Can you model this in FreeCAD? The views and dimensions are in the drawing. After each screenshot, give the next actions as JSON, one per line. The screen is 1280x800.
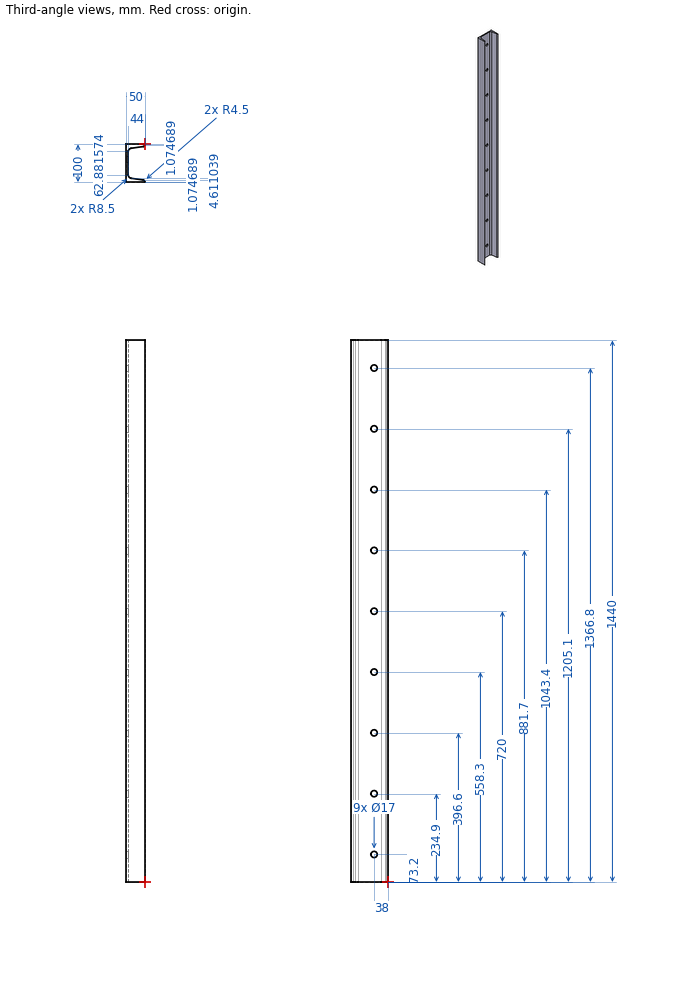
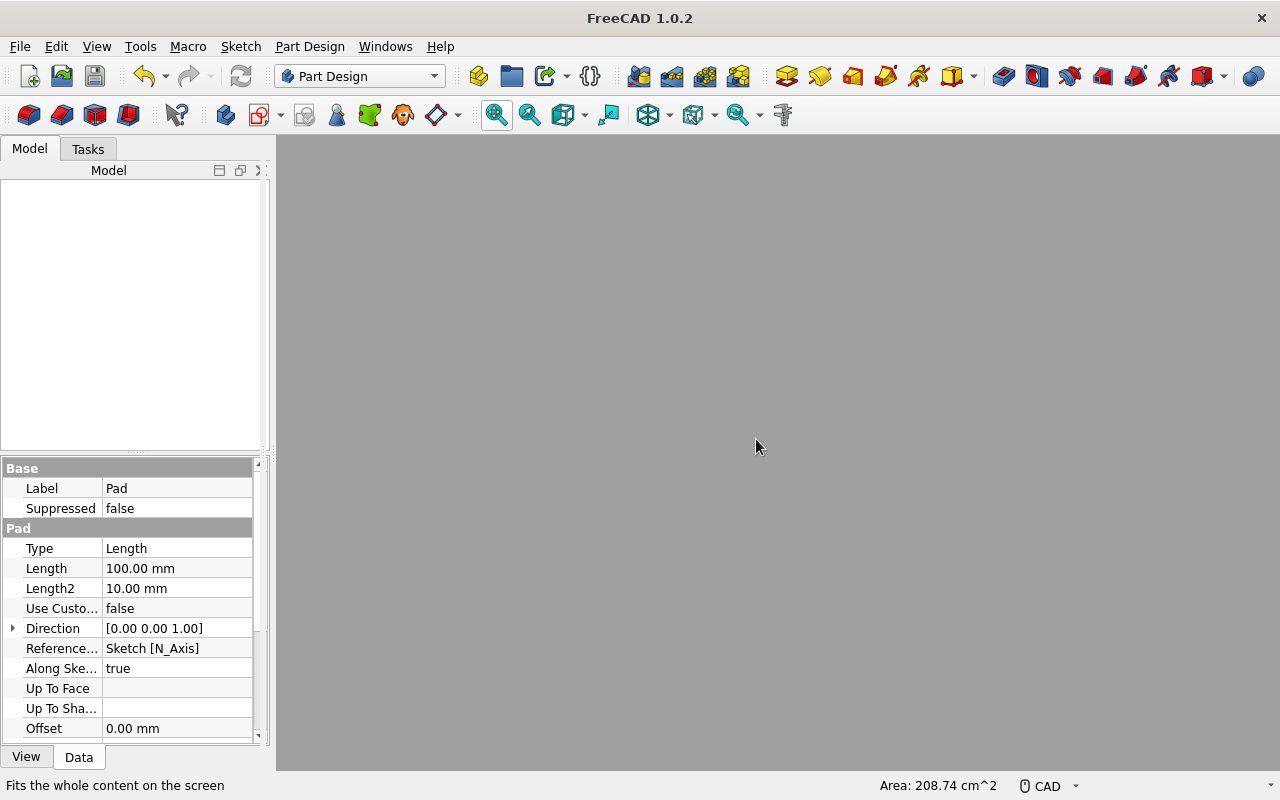
{"action": "left_click", "coordinate": [29, 76]}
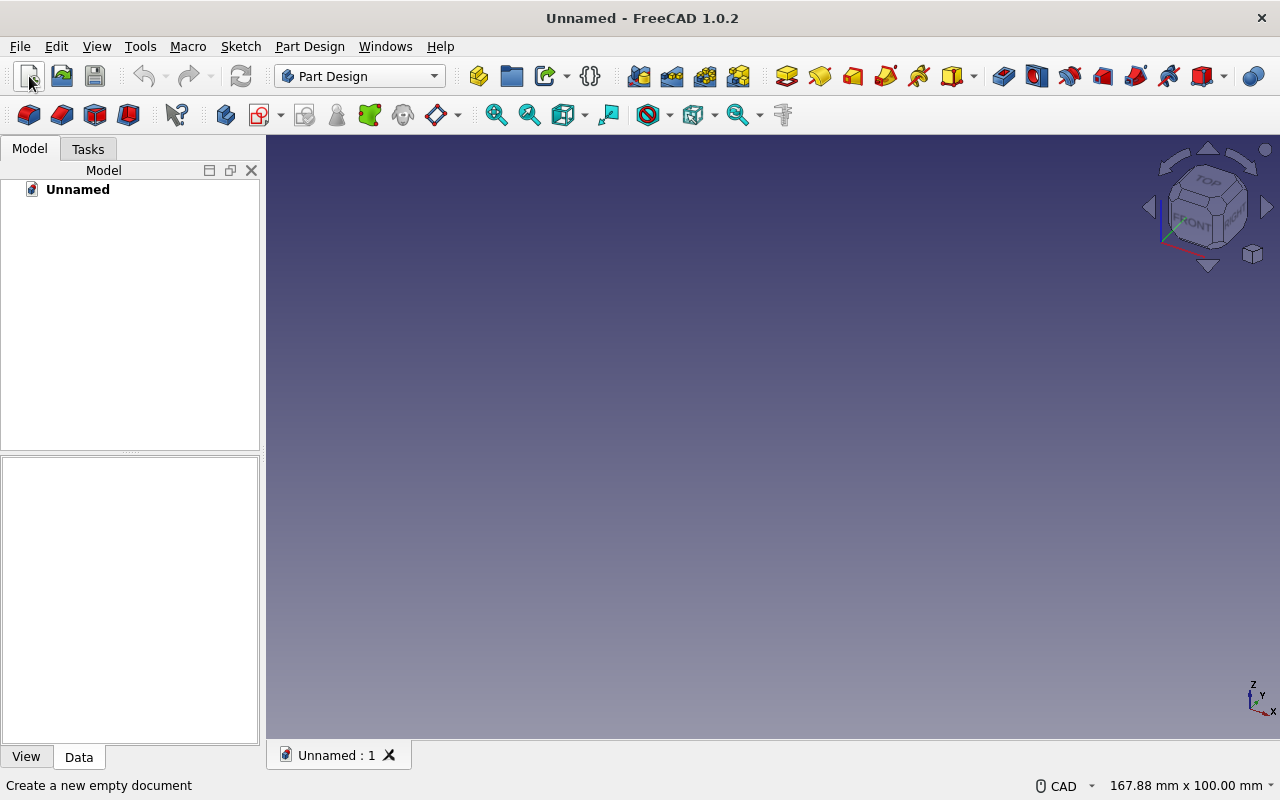
{"action": "left_click", "coordinate": [258, 116]}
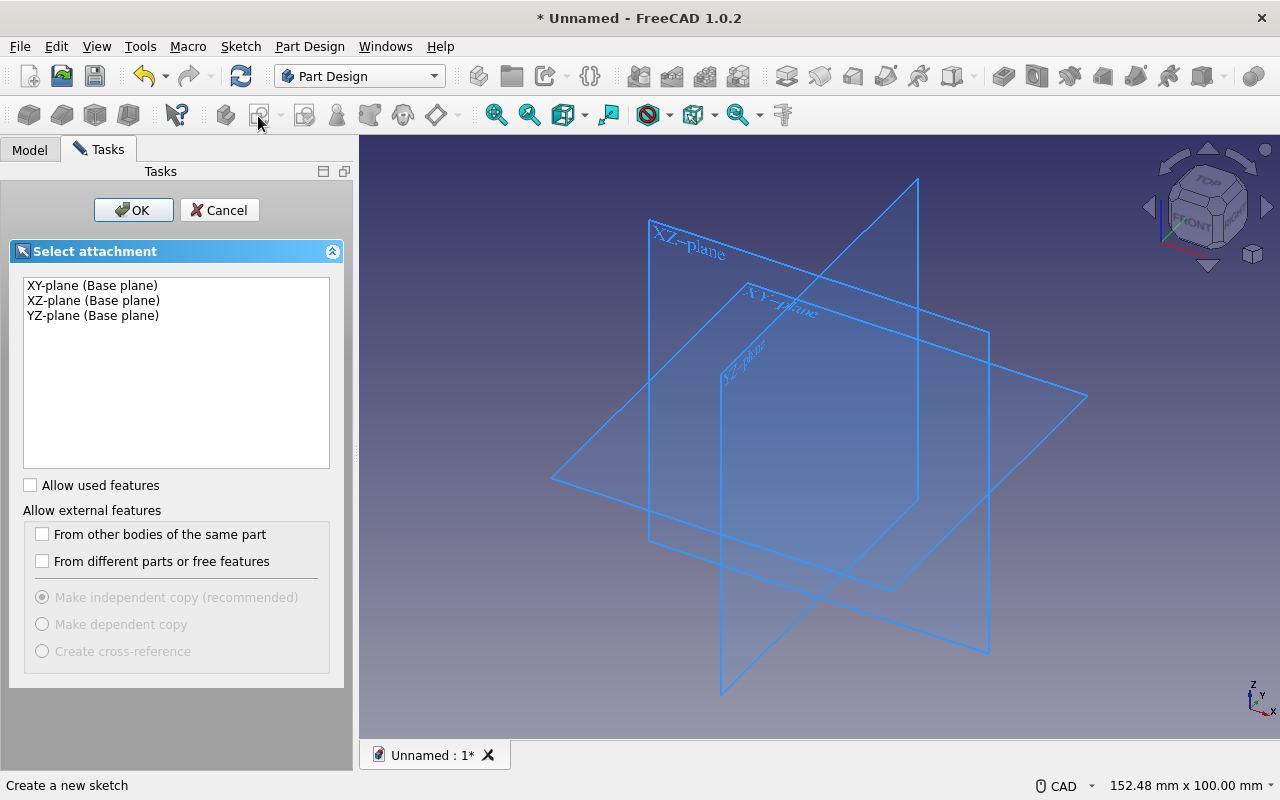
{"action": "left_click", "coordinate": [84, 286]}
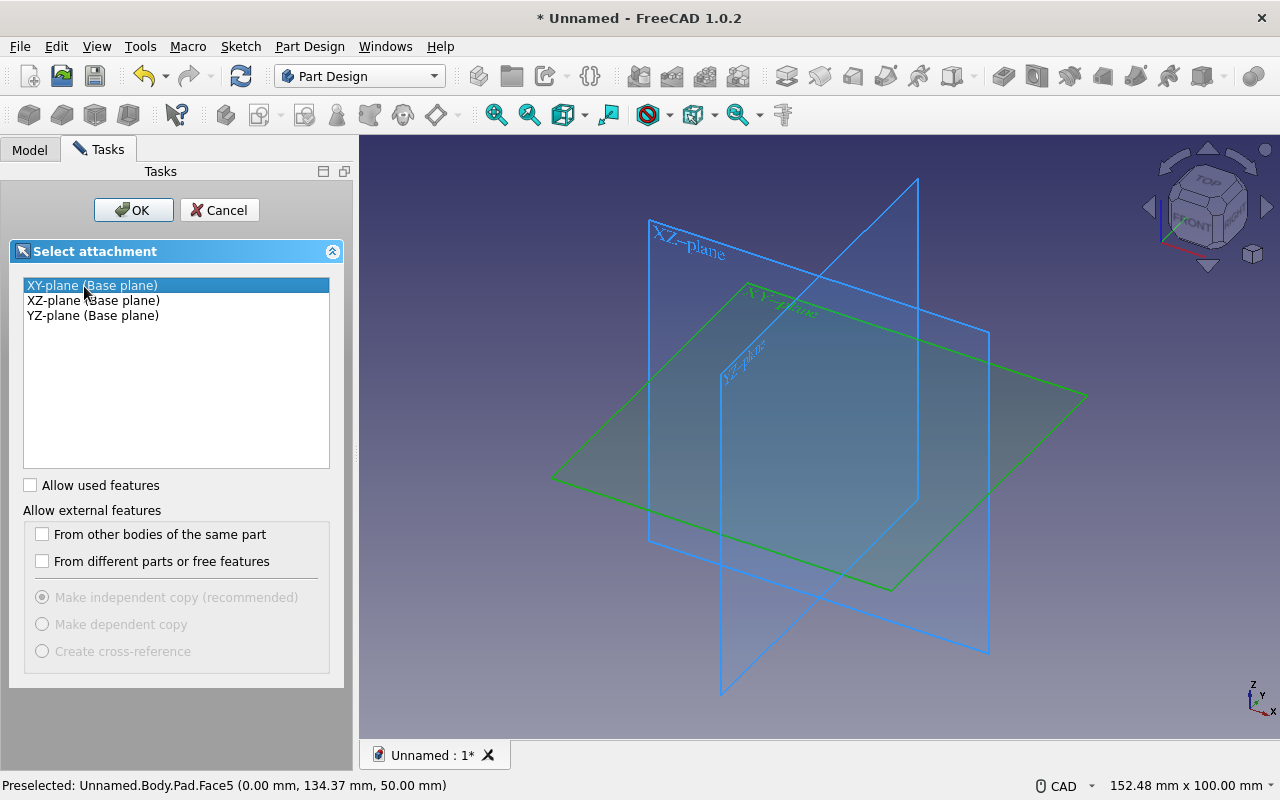
{"action": "left_click", "coordinate": [134, 210]}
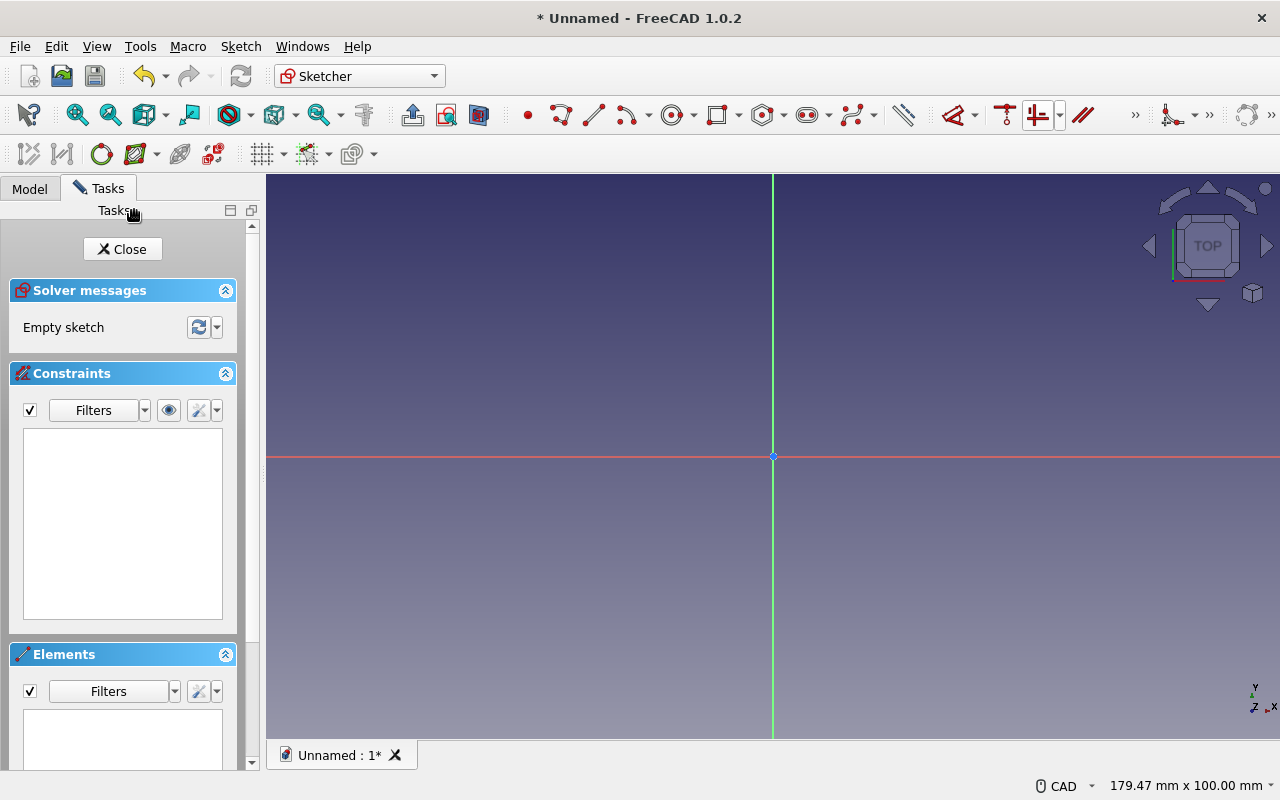
{"action": "scroll", "coordinate": [793, 202], "scroll_direction": "down", "scroll_amount": 3}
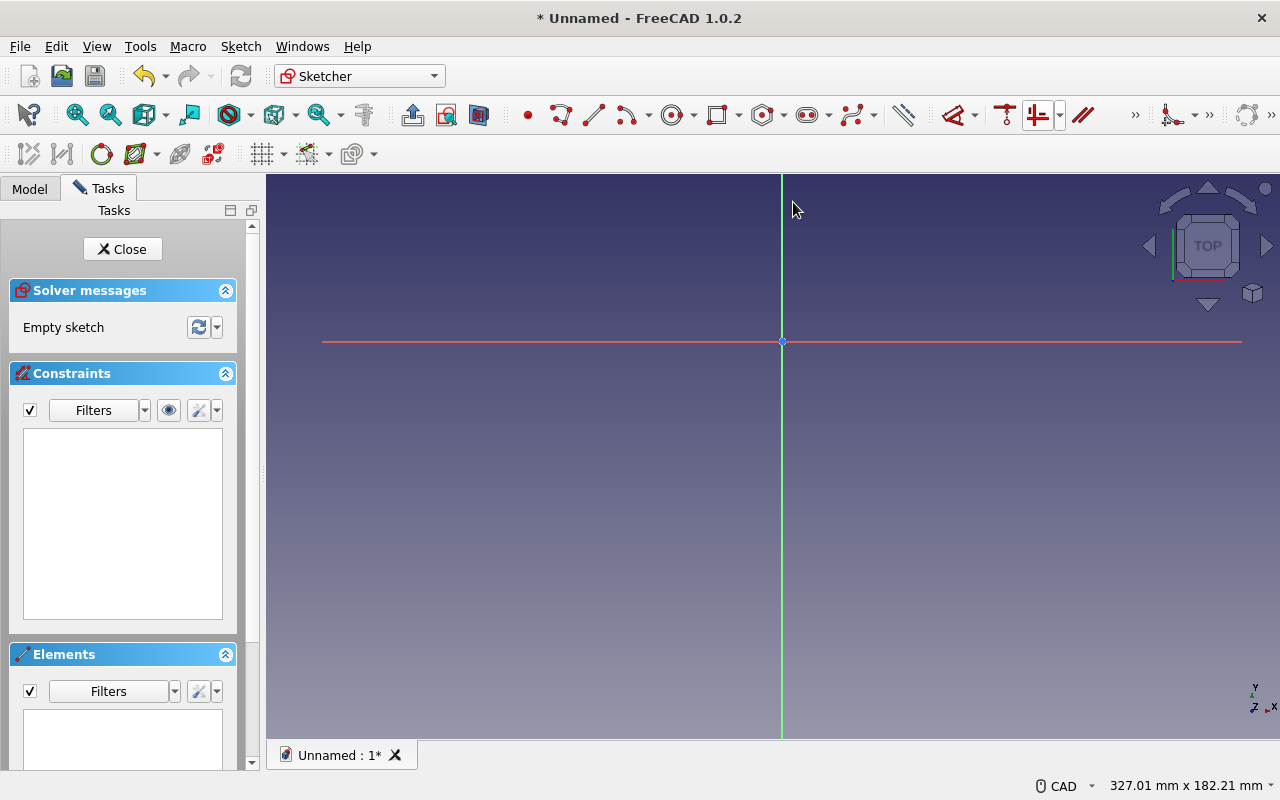
{"action": "left_click", "coordinate": [594, 116]}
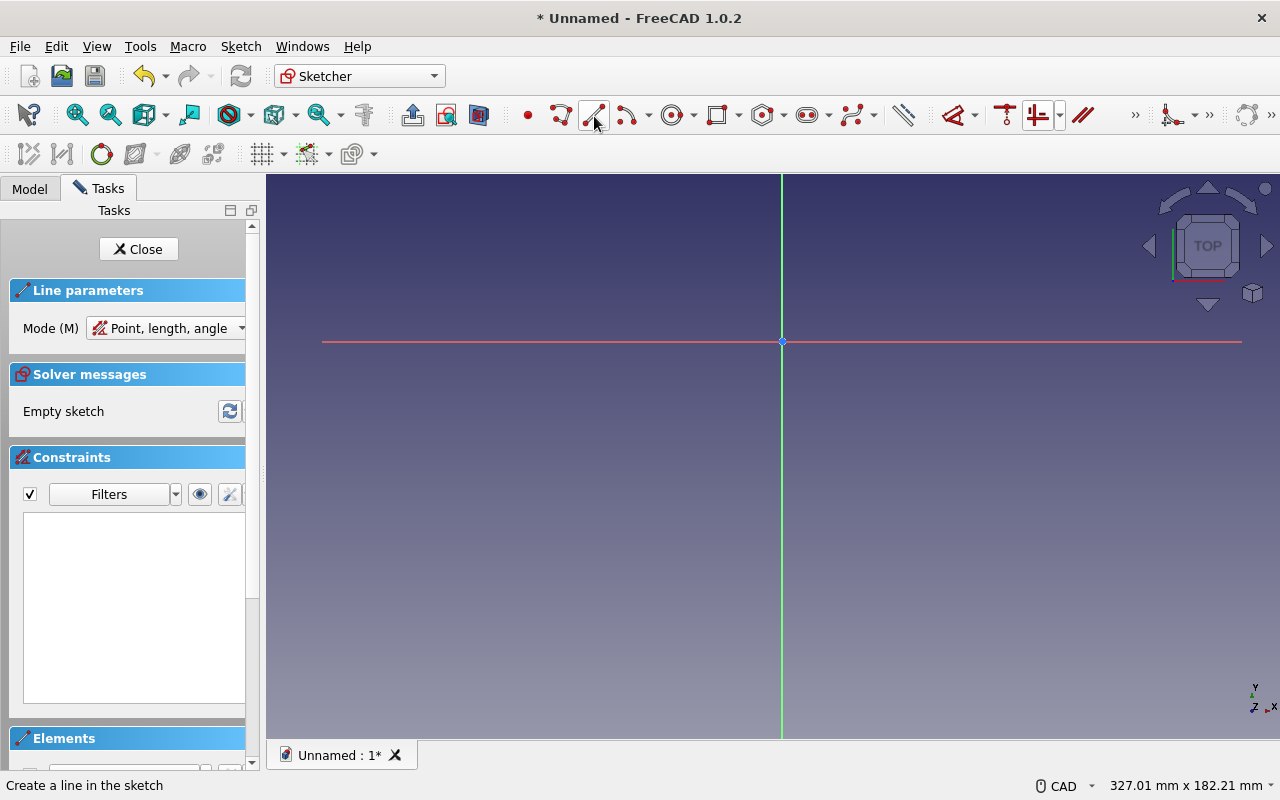
{"action": "scroll", "coordinate": [770, 635], "scroll_direction": "up", "scroll_amount": 2}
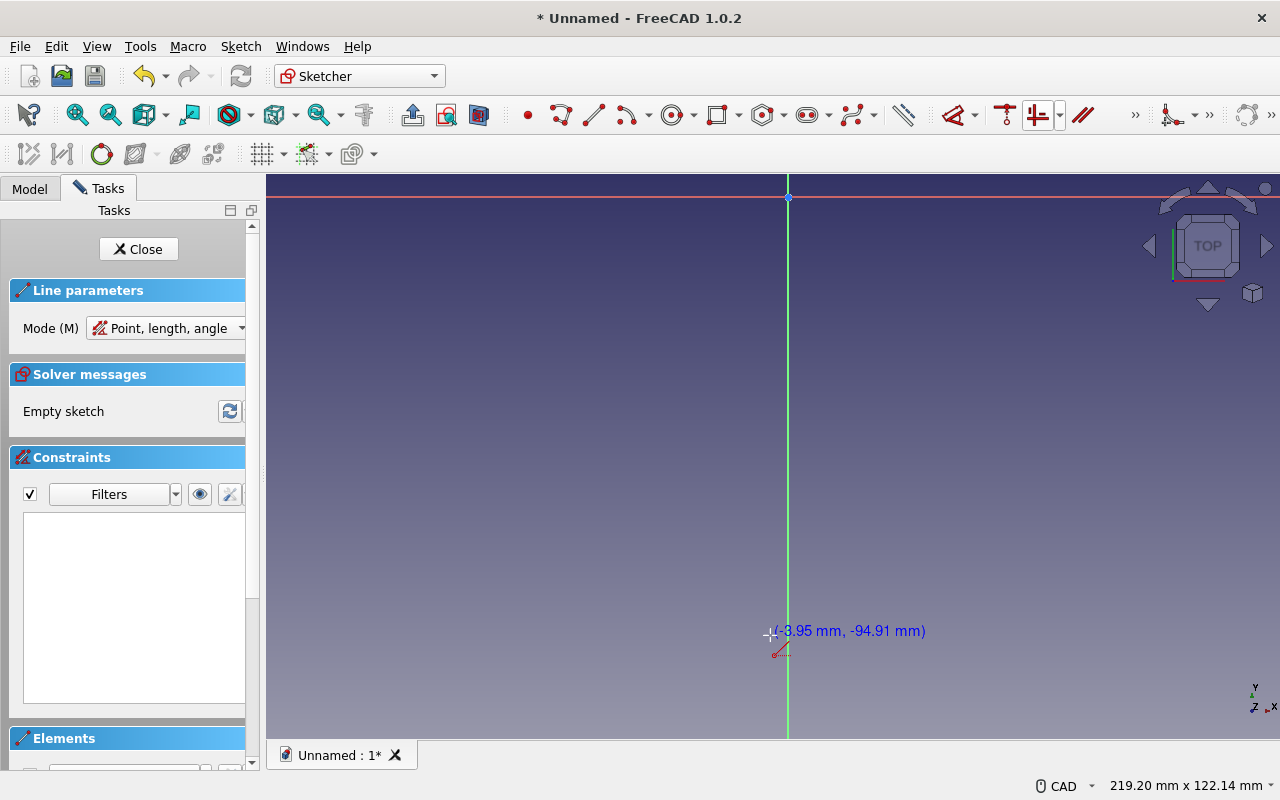
{"action": "left_click", "coordinate": [770, 634]}
{"action": "left_click", "coordinate": [618, 613]}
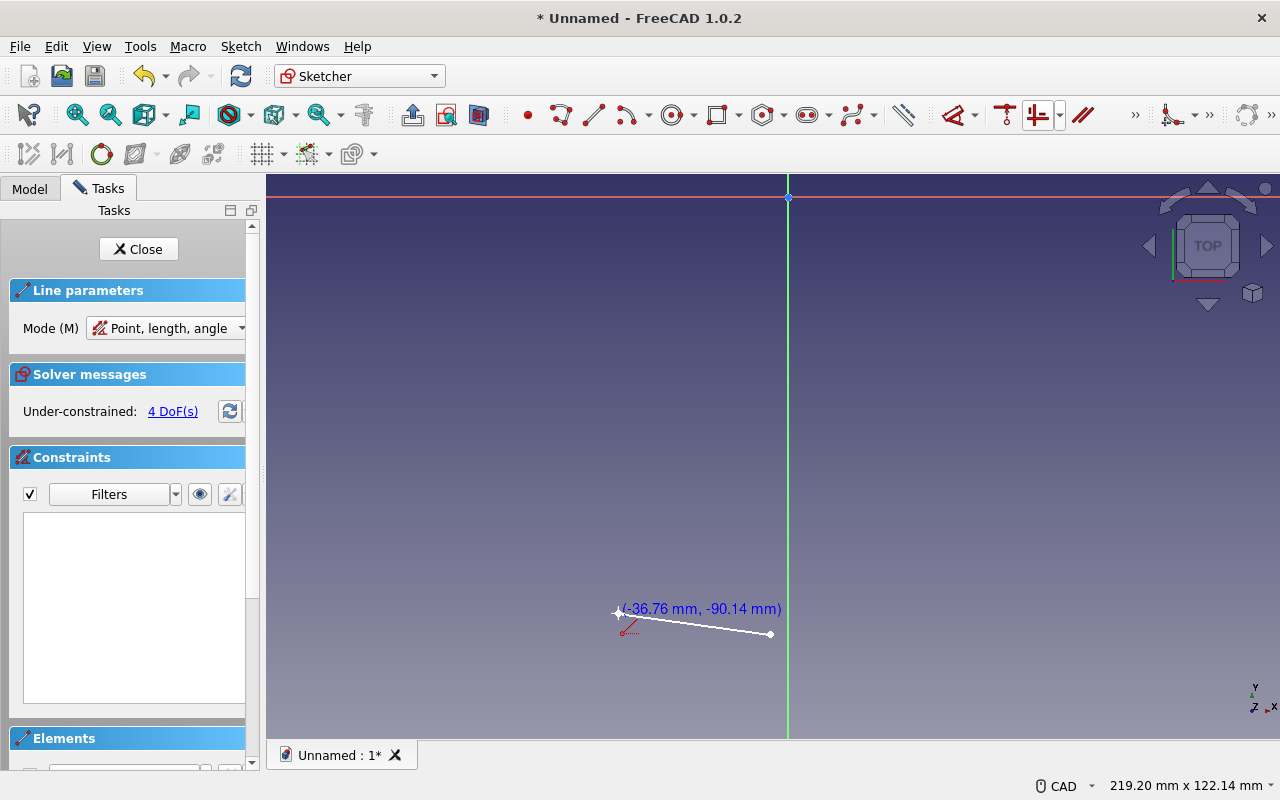
{"action": "left_click", "coordinate": [585, 574]}
{"action": "left_click", "coordinate": [585, 283]}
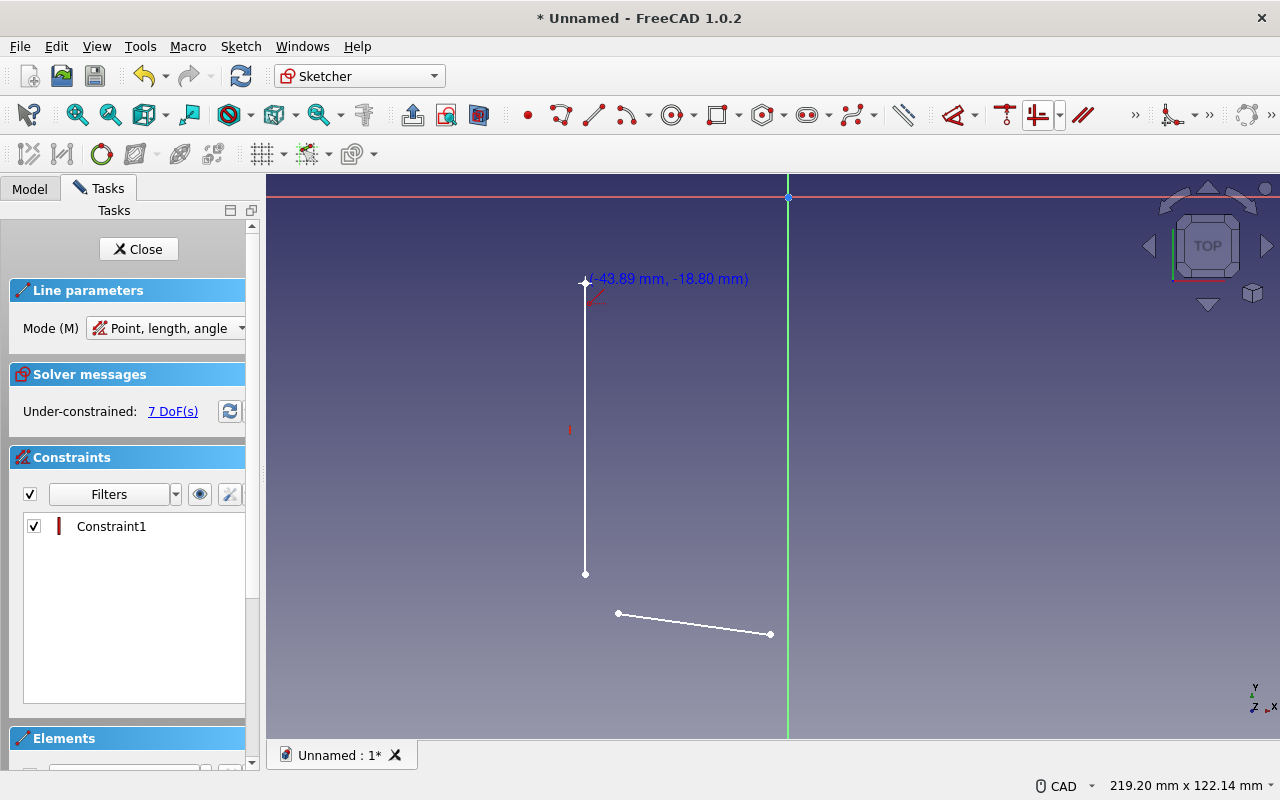
{"action": "left_click", "coordinate": [618, 244]}
{"action": "left_click", "coordinate": [770, 223]}